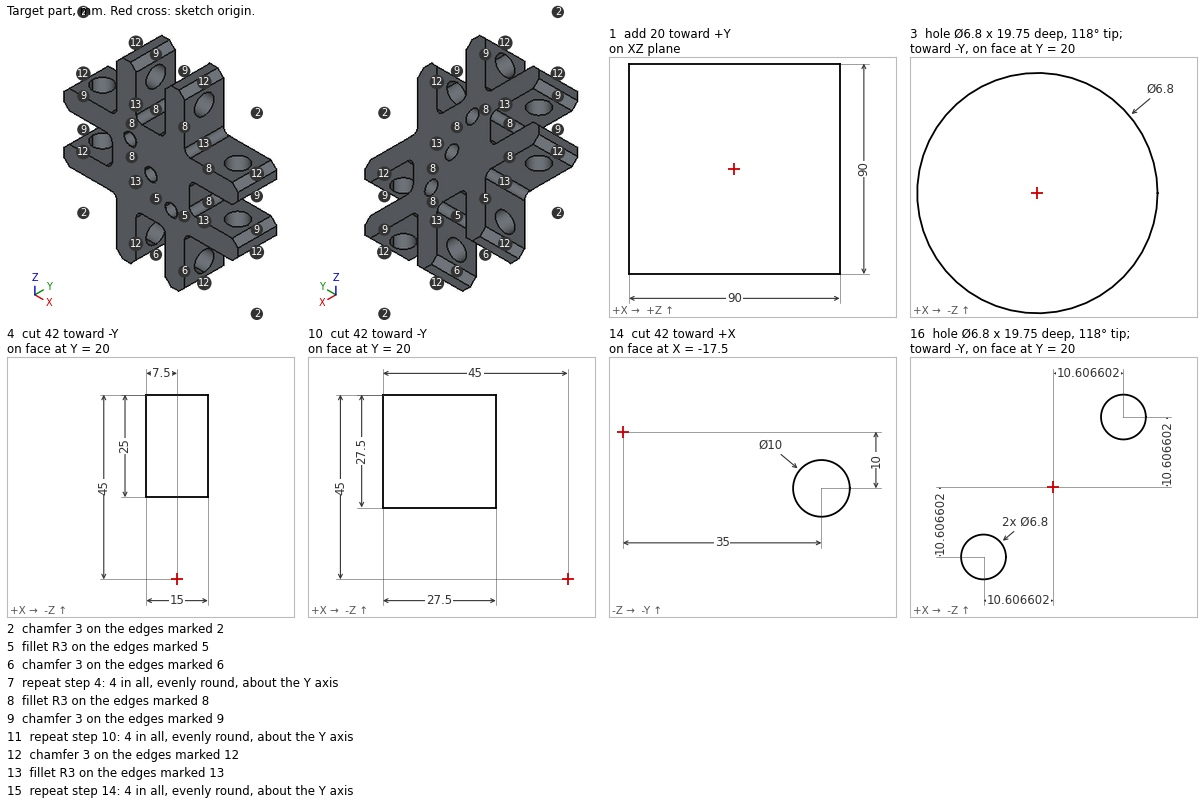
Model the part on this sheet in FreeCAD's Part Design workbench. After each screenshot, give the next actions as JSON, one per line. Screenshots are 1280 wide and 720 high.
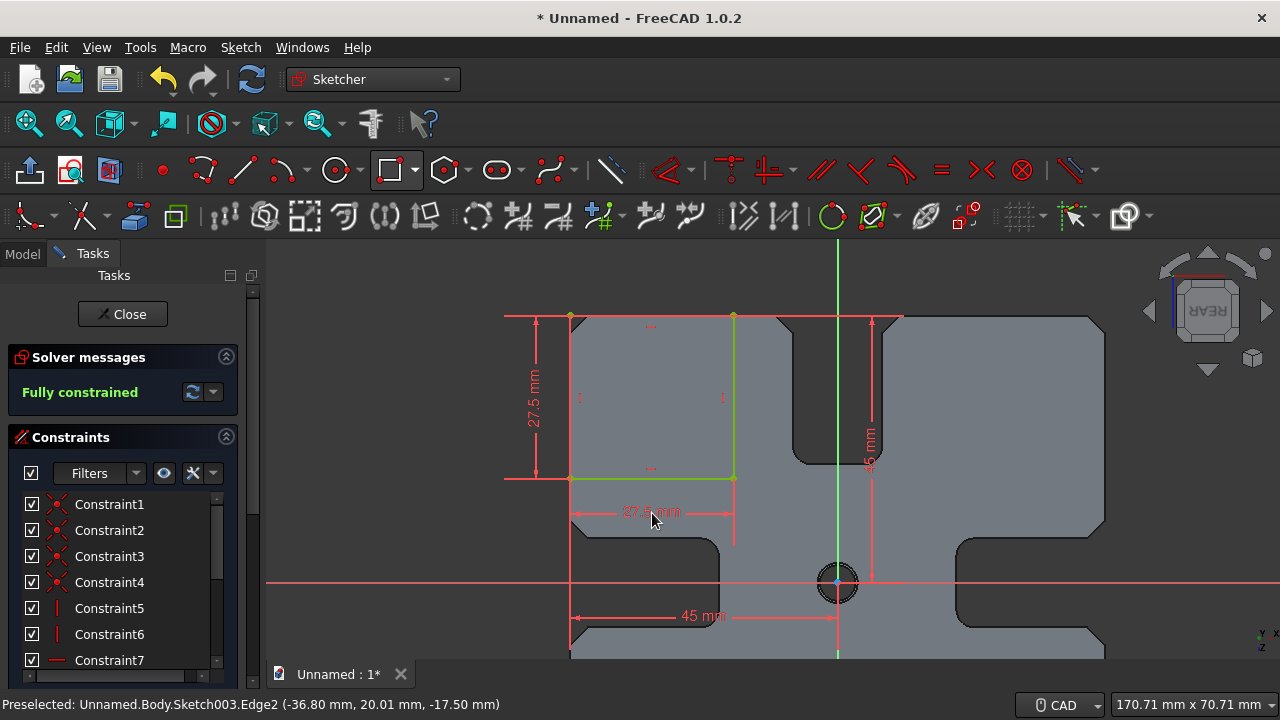
{"action": "left_click", "coordinate": [123, 314]}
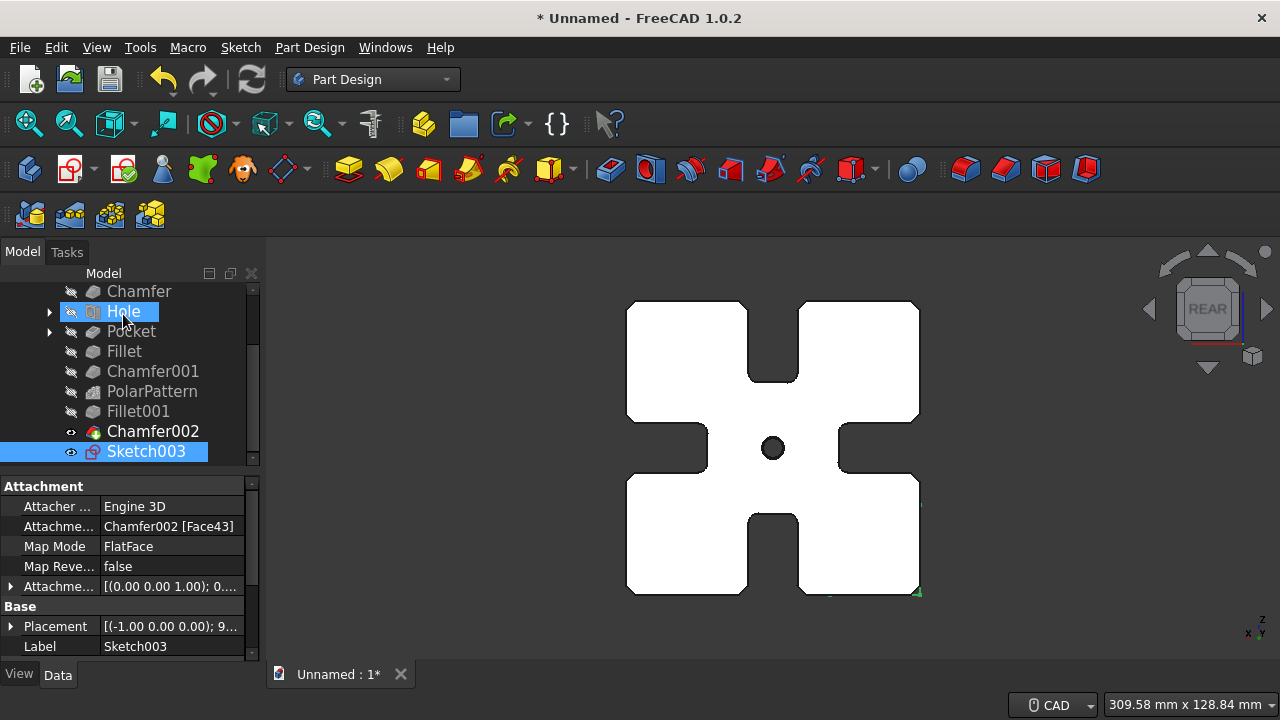
{"action": "left_click", "coordinate": [612, 170]}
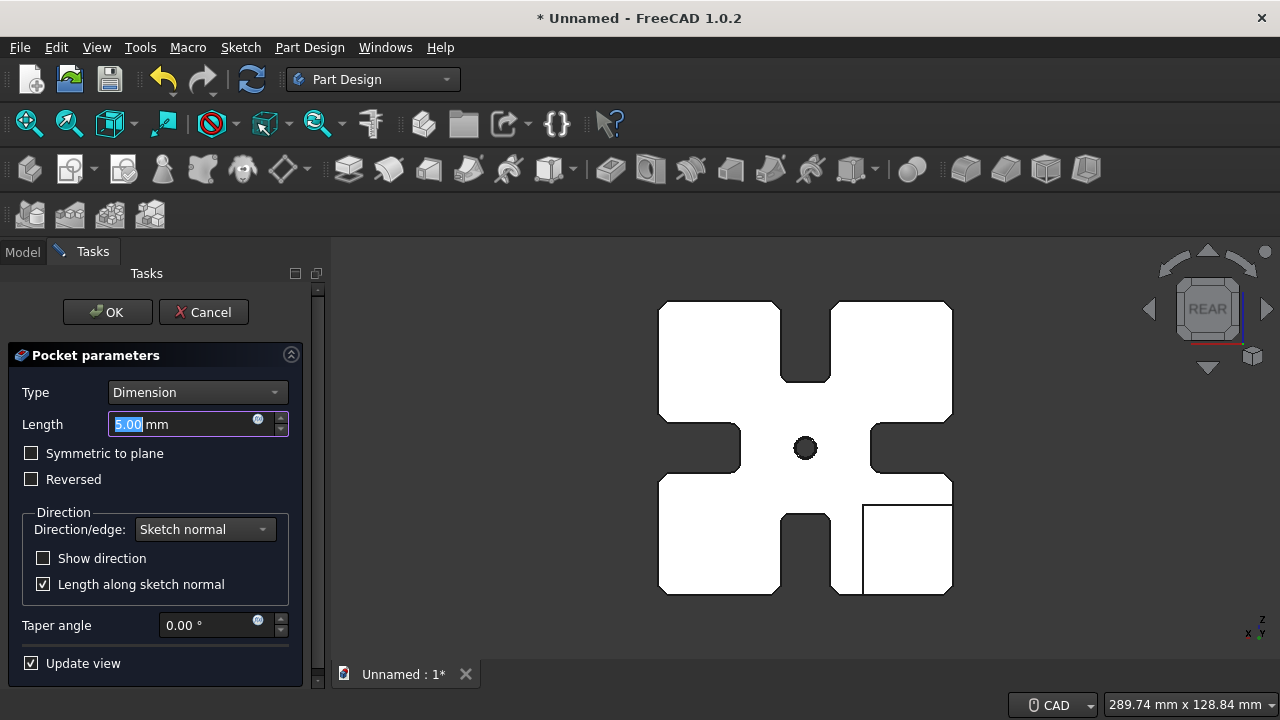
{"action": "type", "text": "42"}
{"action": "key", "text": "Tab"}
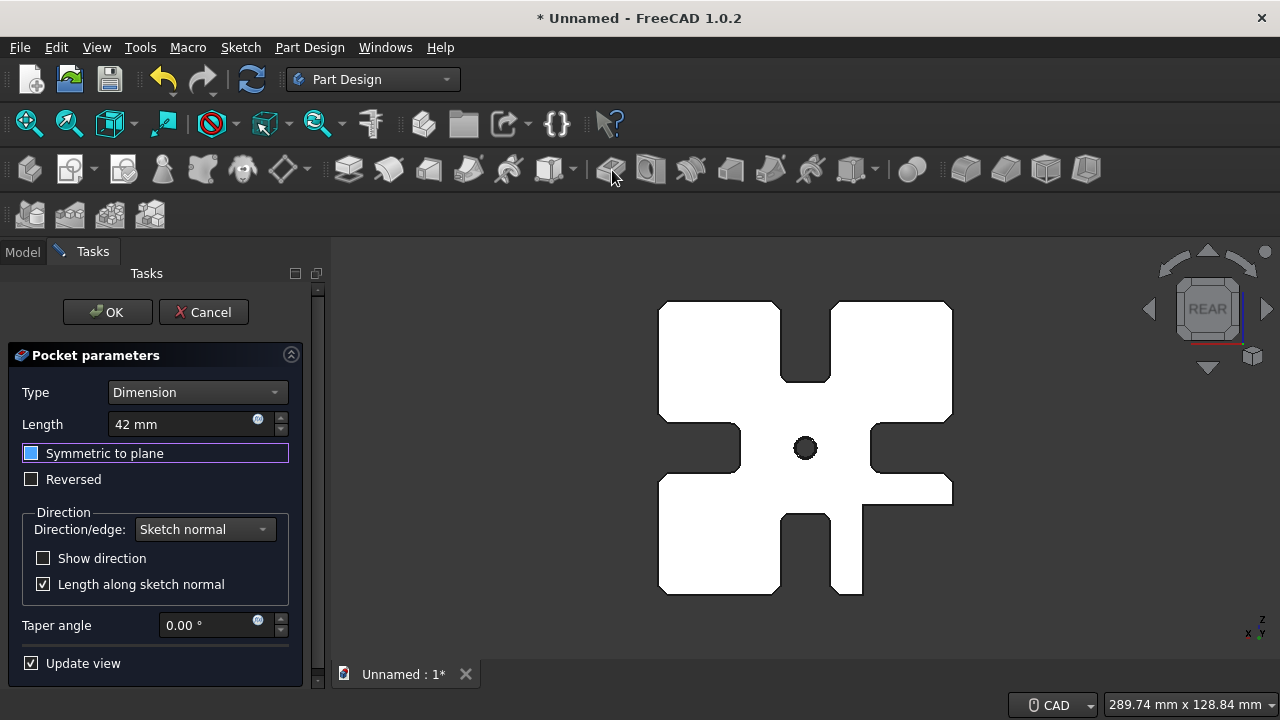
{"action": "left_click", "coordinate": [108, 312]}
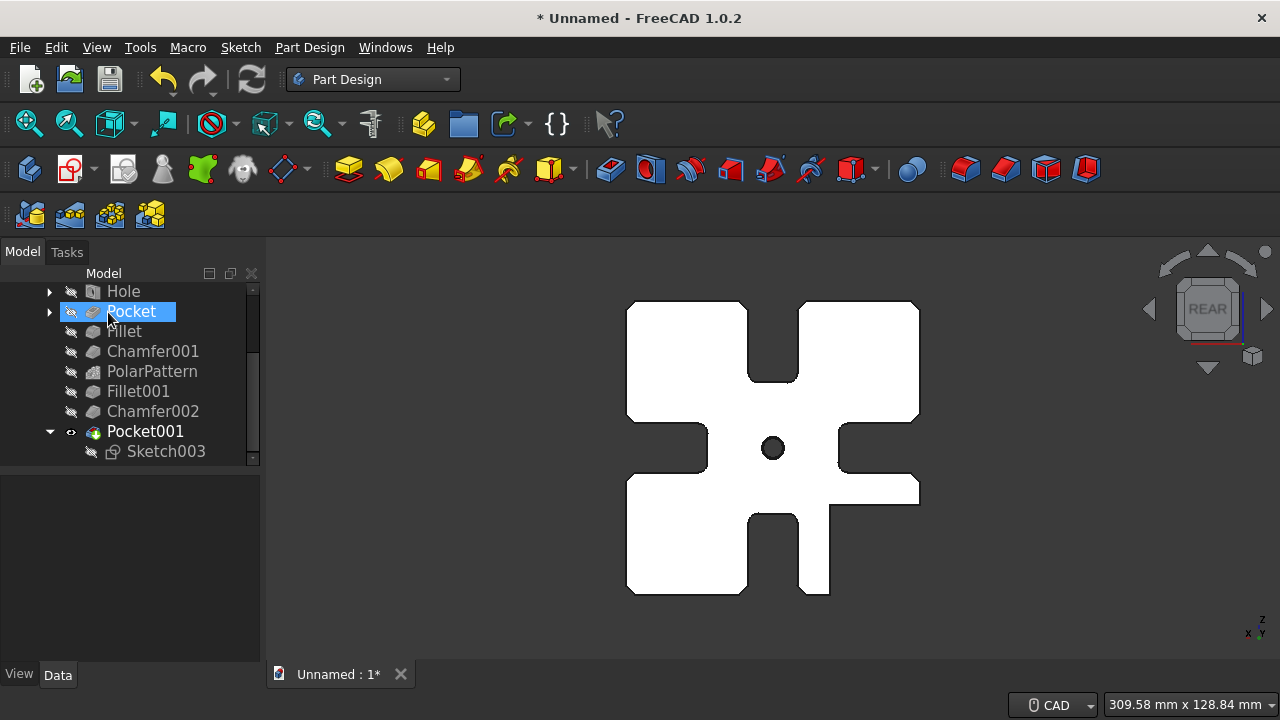
{"action": "left_click", "coordinate": [116, 432]}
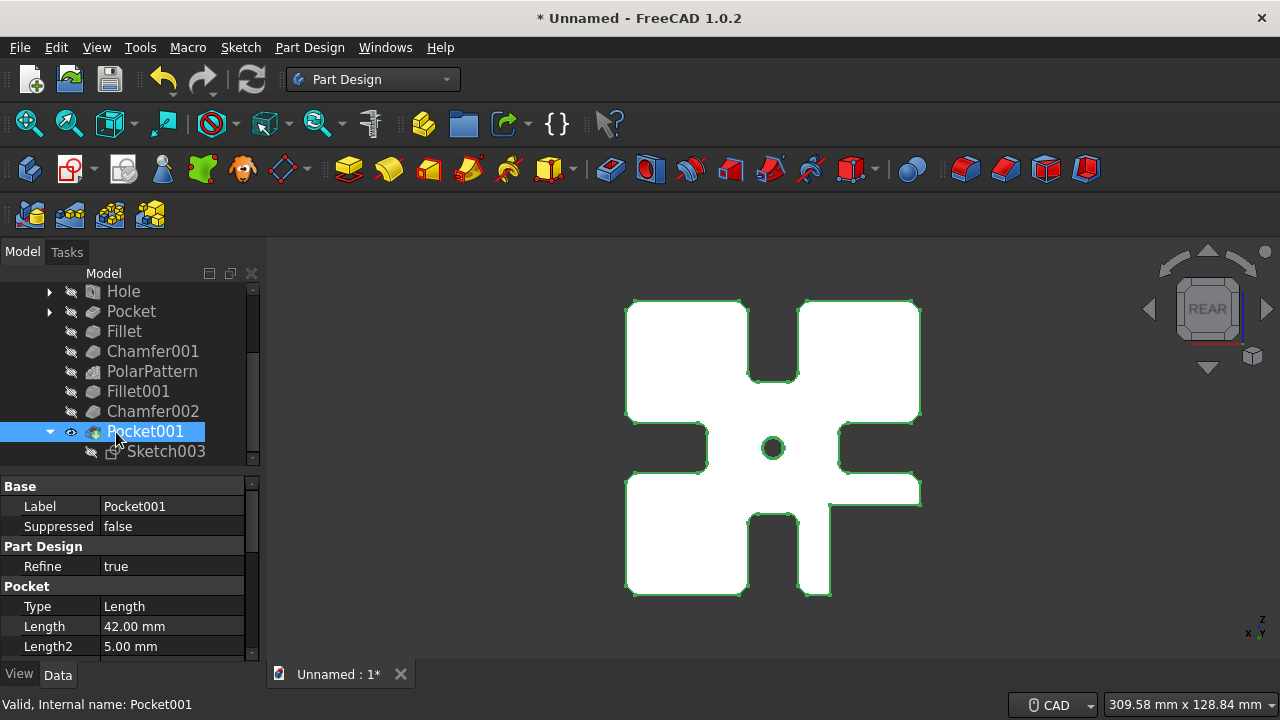
{"action": "left_click", "coordinate": [110, 214]}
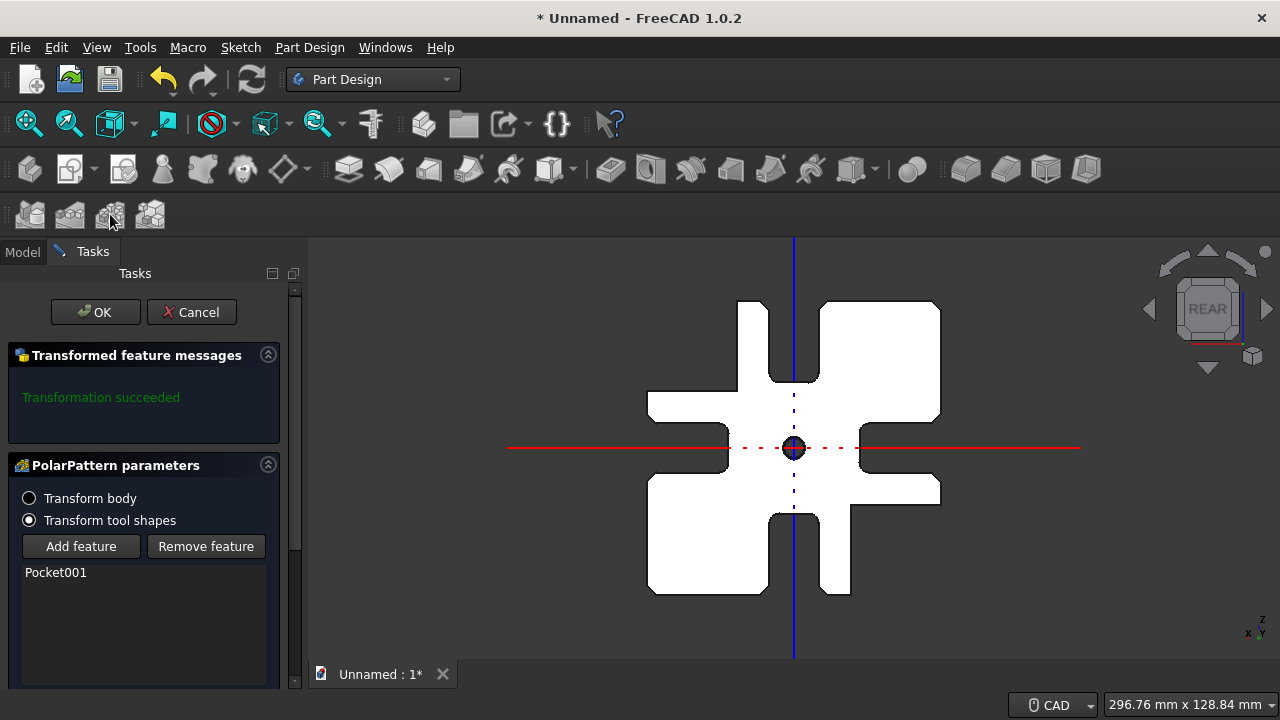
{"action": "scroll", "coordinate": [295, 486], "scroll_direction": "down", "scroll_amount": 2}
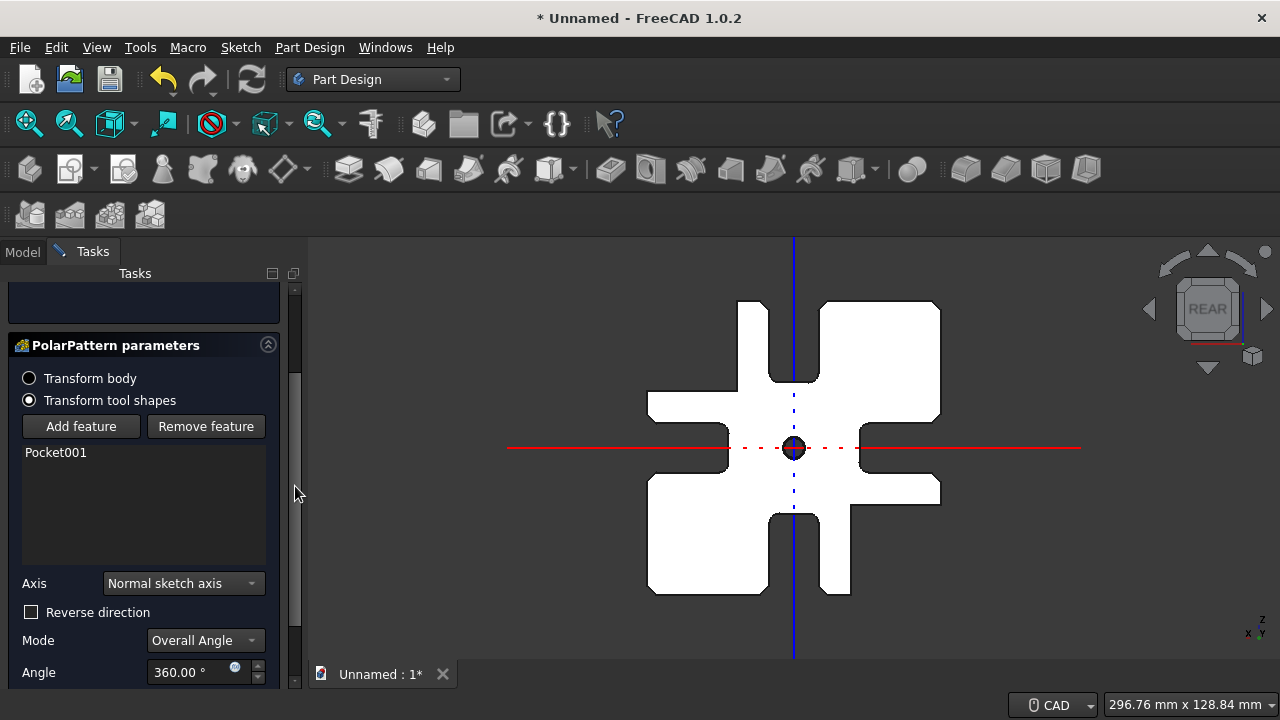
{"action": "left_click", "coordinate": [184, 584]}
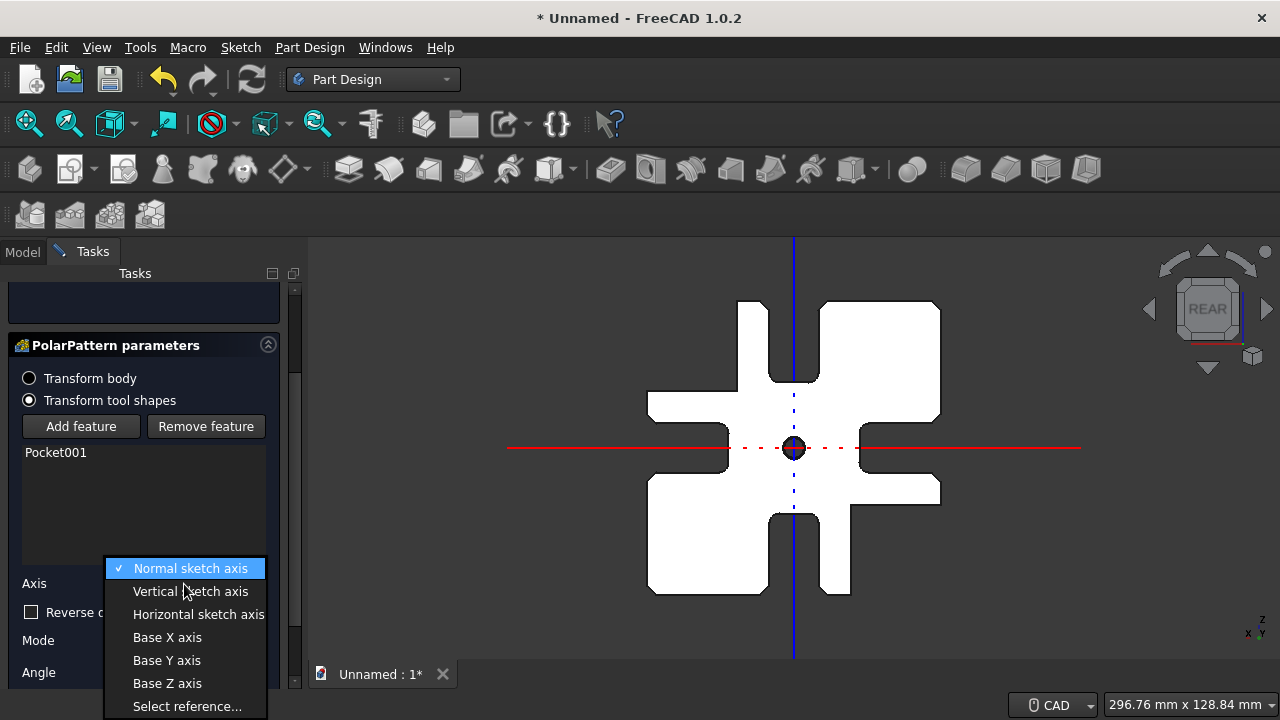
{"action": "left_click", "coordinate": [184, 660]}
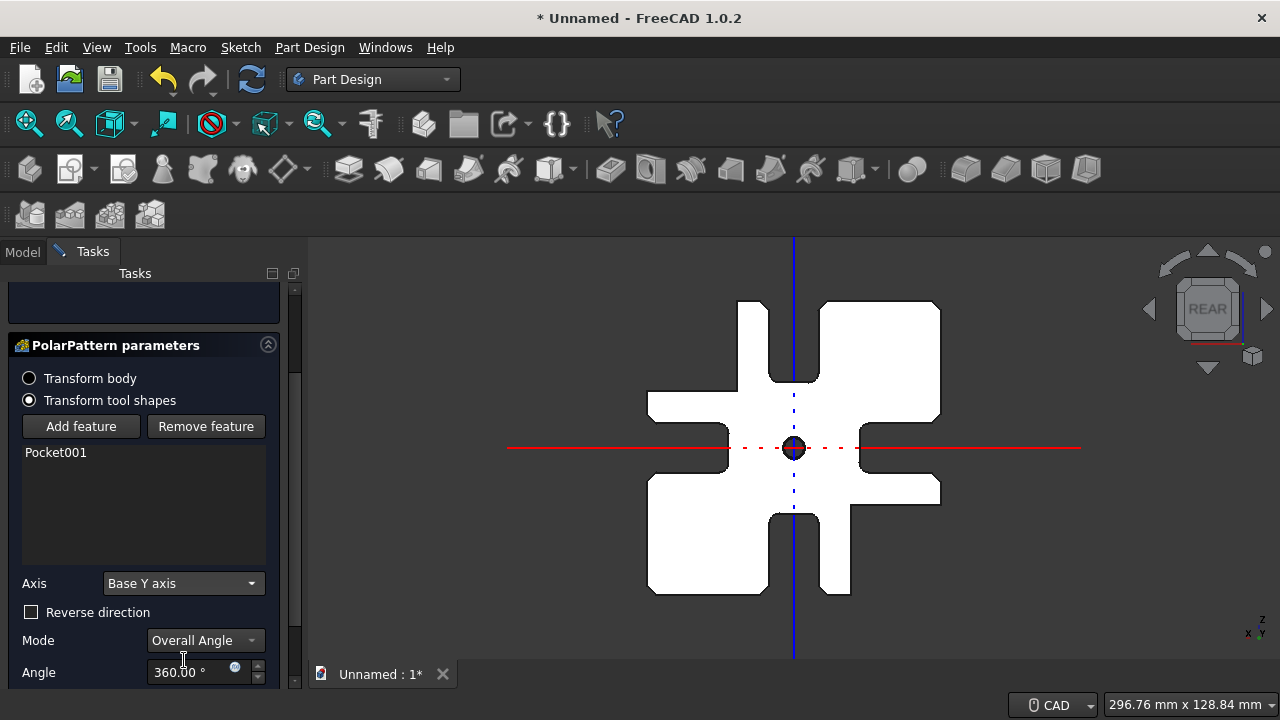
{"action": "scroll", "coordinate": [295, 486], "scroll_direction": "down", "scroll_amount": 2}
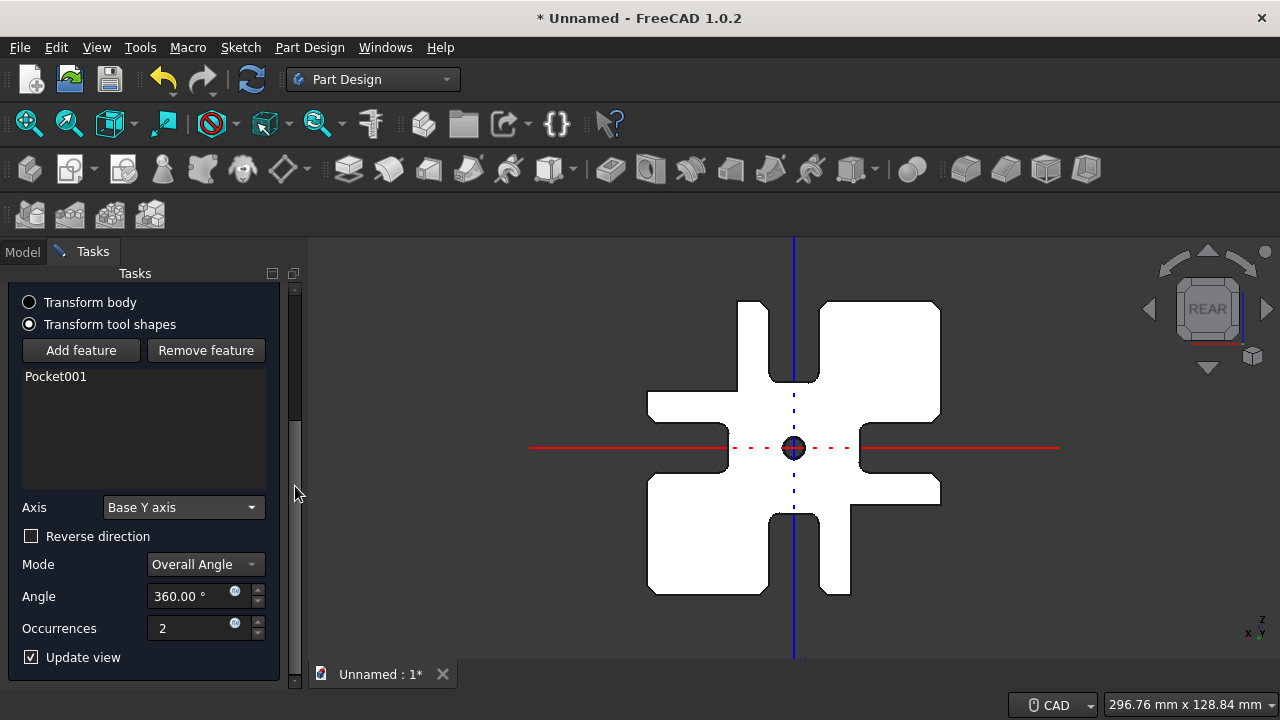
{"action": "triple_click", "coordinate": [198, 628]}